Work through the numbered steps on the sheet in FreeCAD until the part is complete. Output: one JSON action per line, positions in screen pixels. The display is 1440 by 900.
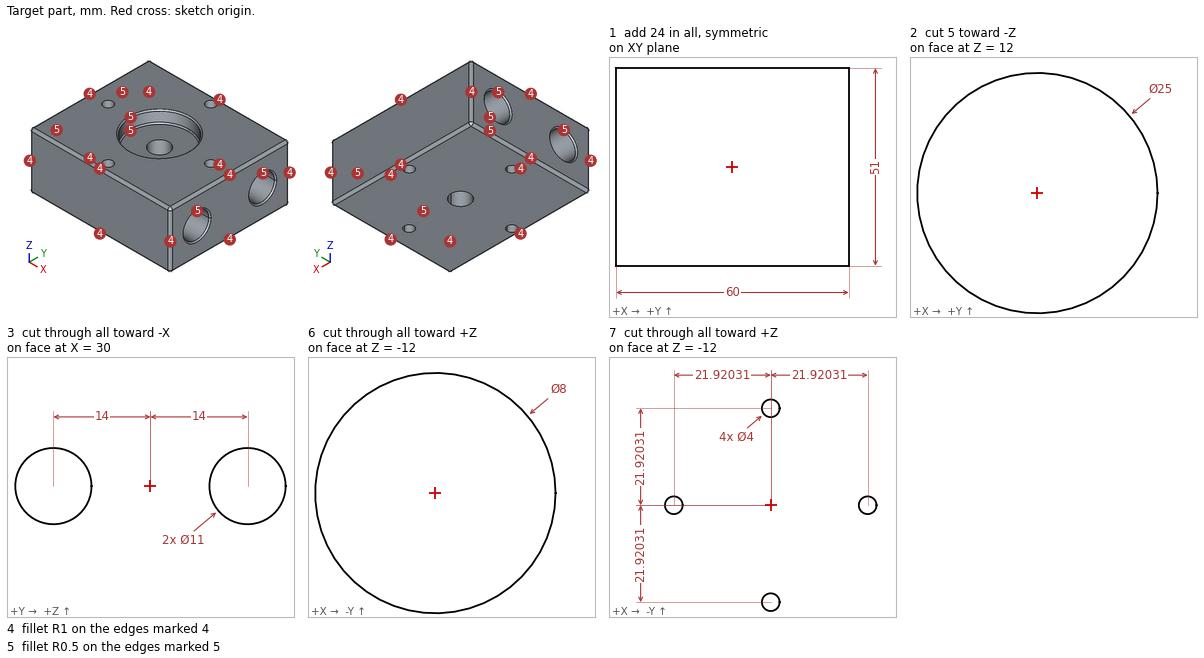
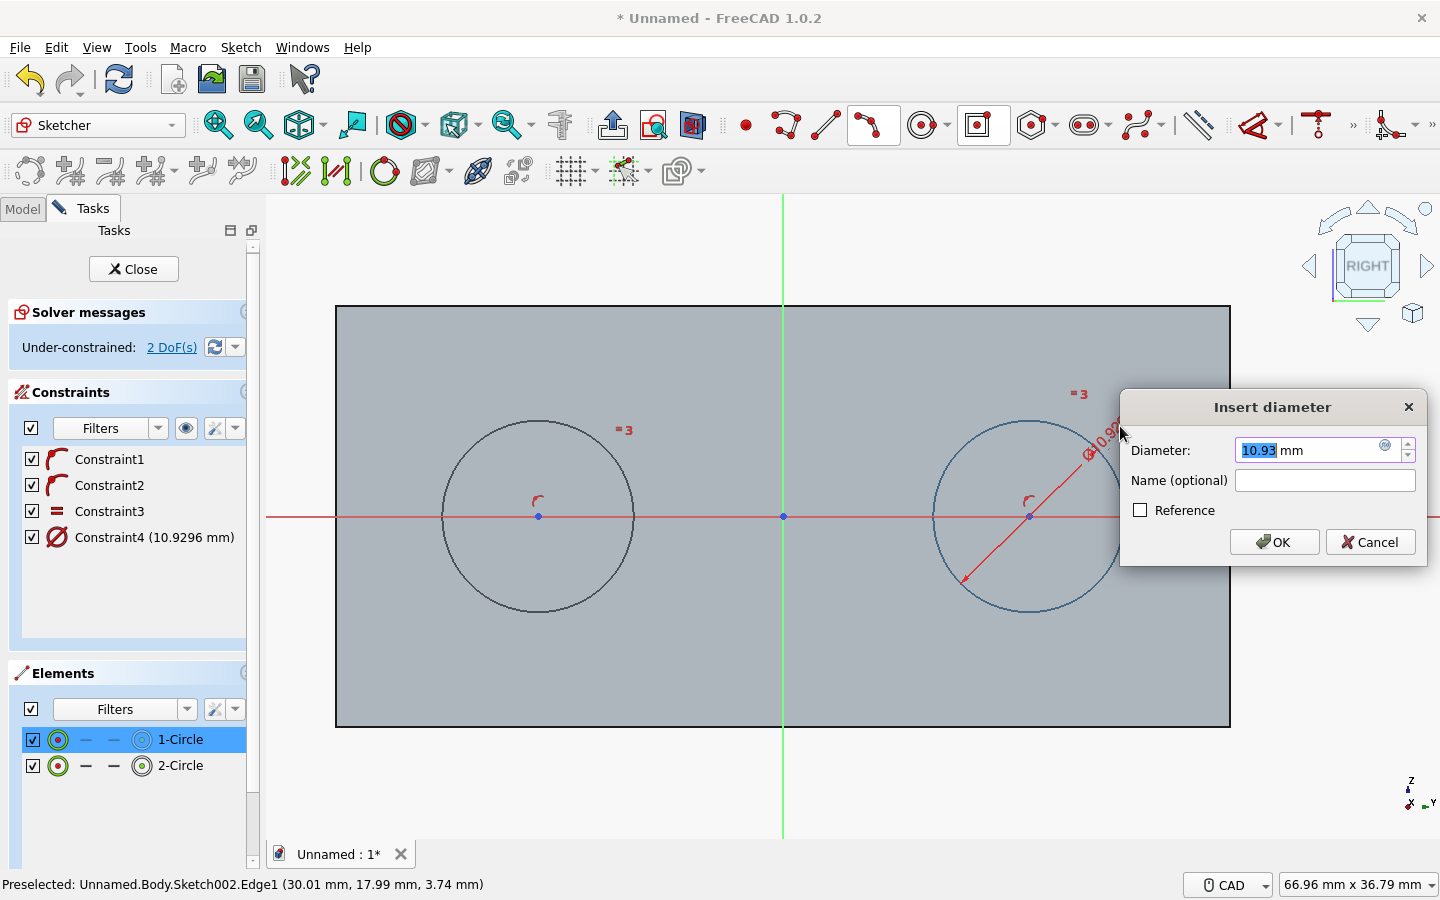
{"action": "type", "text": "11"}
{"action": "key", "text": "Return"}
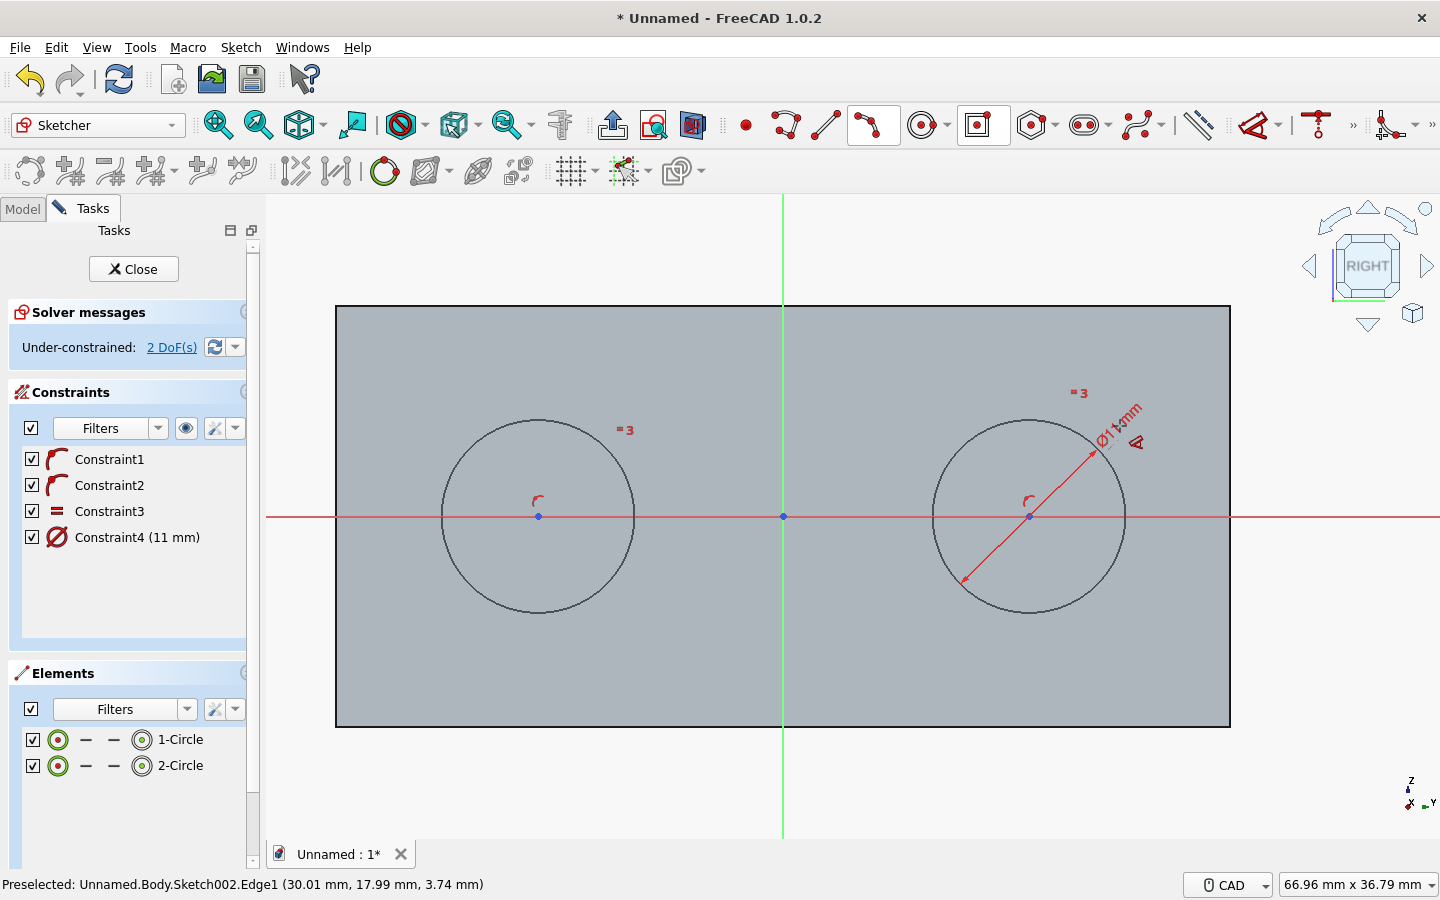
{"action": "left_click", "coordinate": [1029, 516]}
{"action": "left_click", "coordinate": [906, 550]}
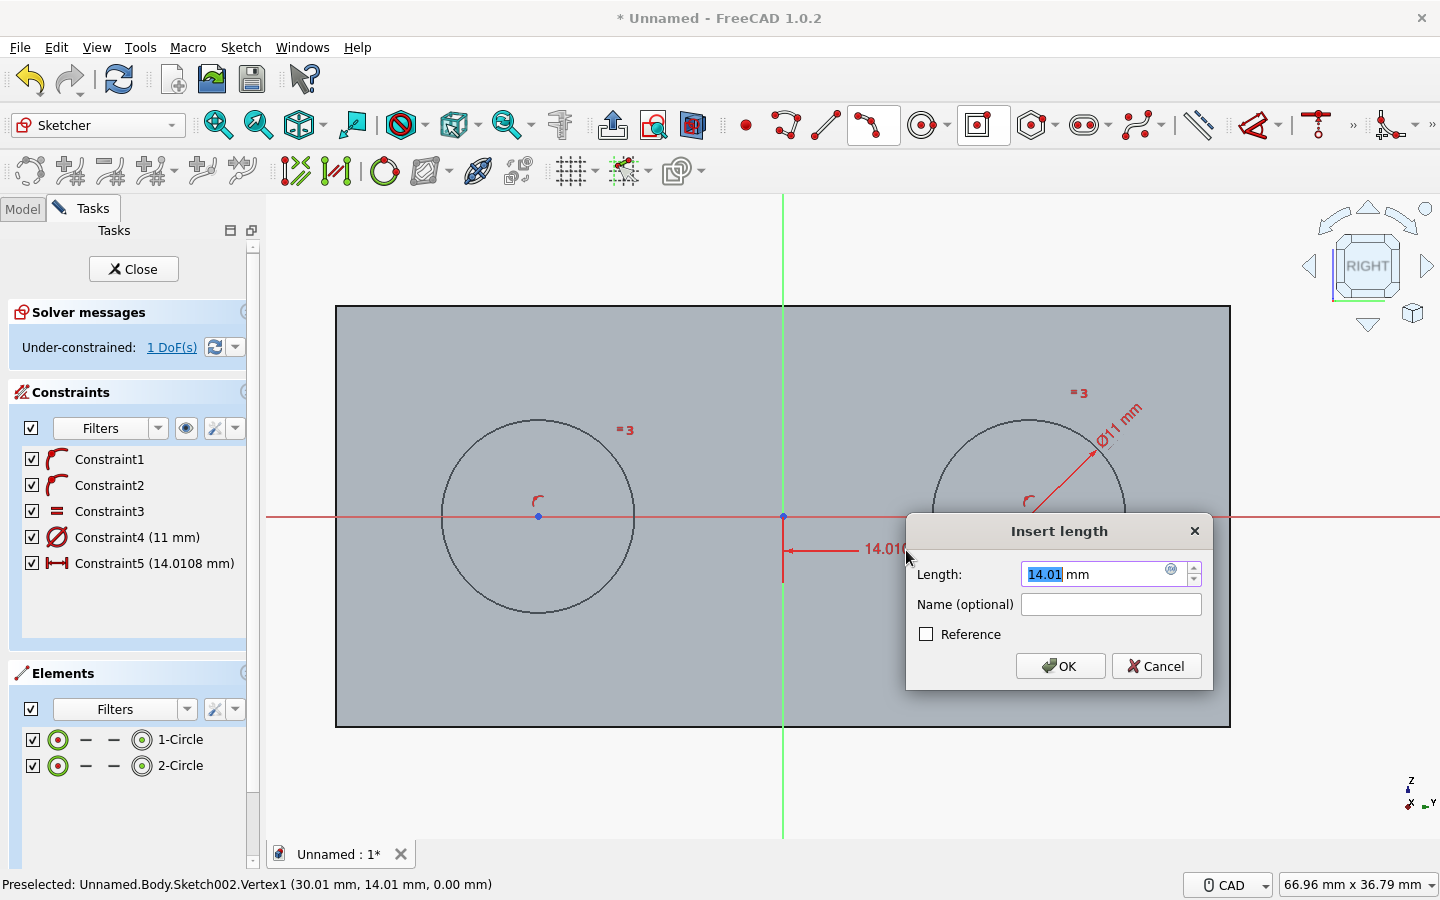
{"action": "type", "text": "14"}
{"action": "key", "text": "Return"}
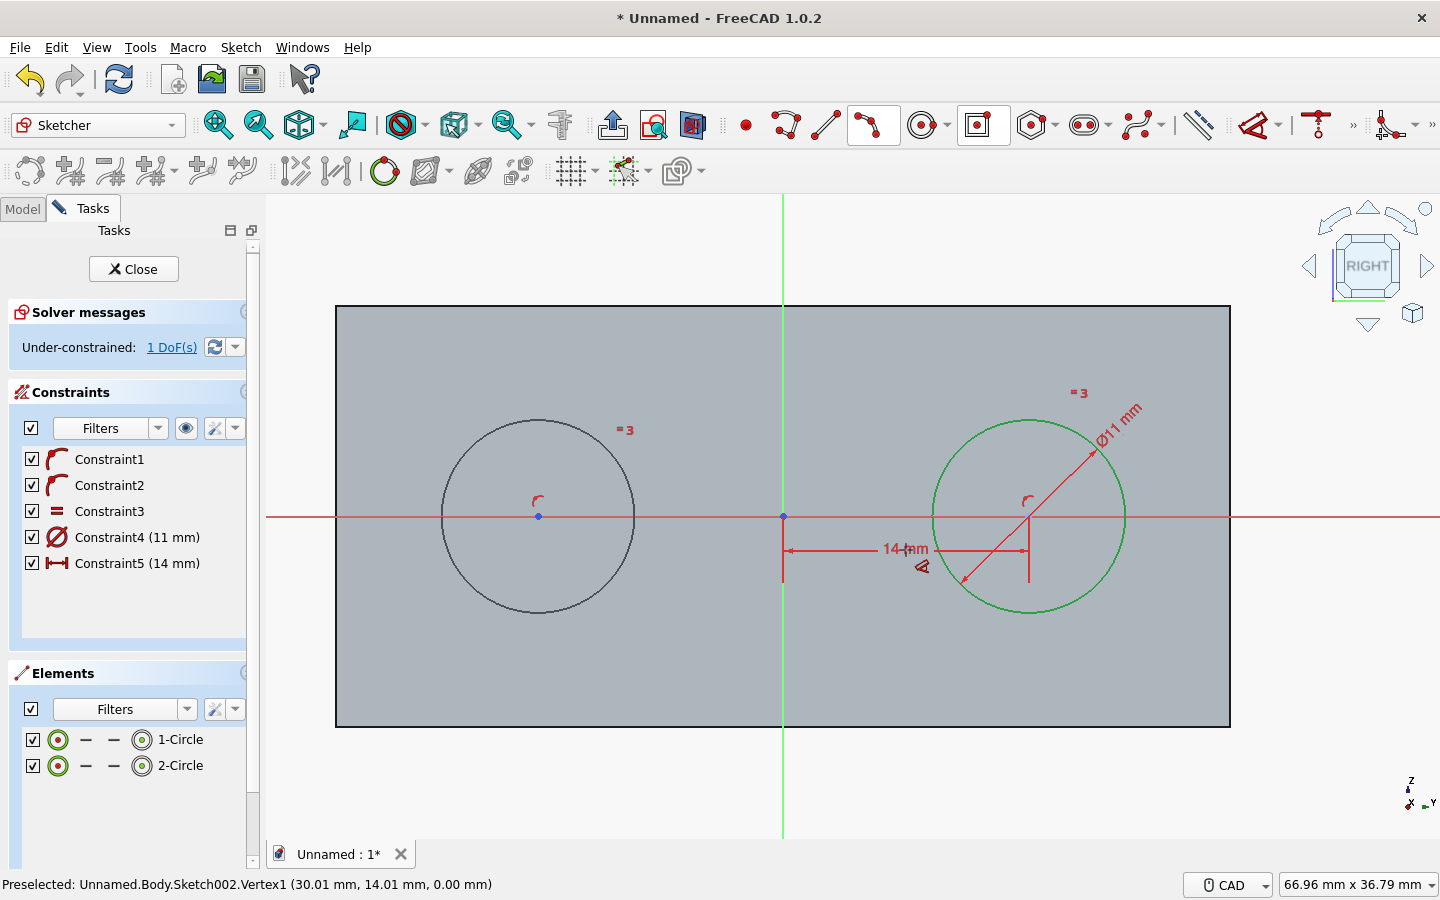
{"action": "left_click", "coordinate": [538, 516]}
{"action": "left_click", "coordinate": [661, 550]}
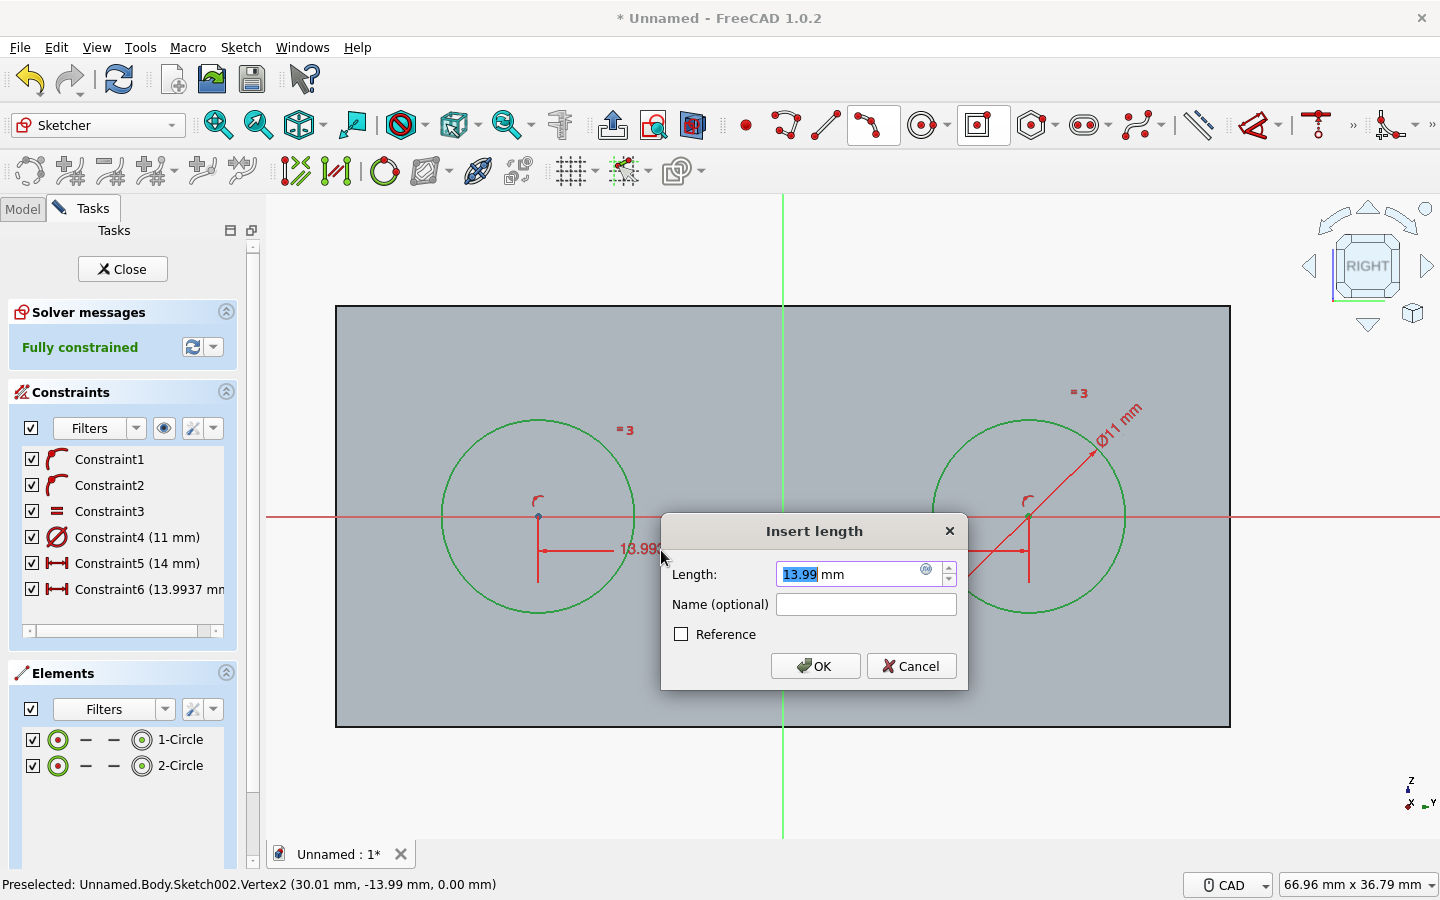
{"action": "type", "text": "14"}
{"action": "key", "text": "Return"}
{"action": "key", "text": "Escape"}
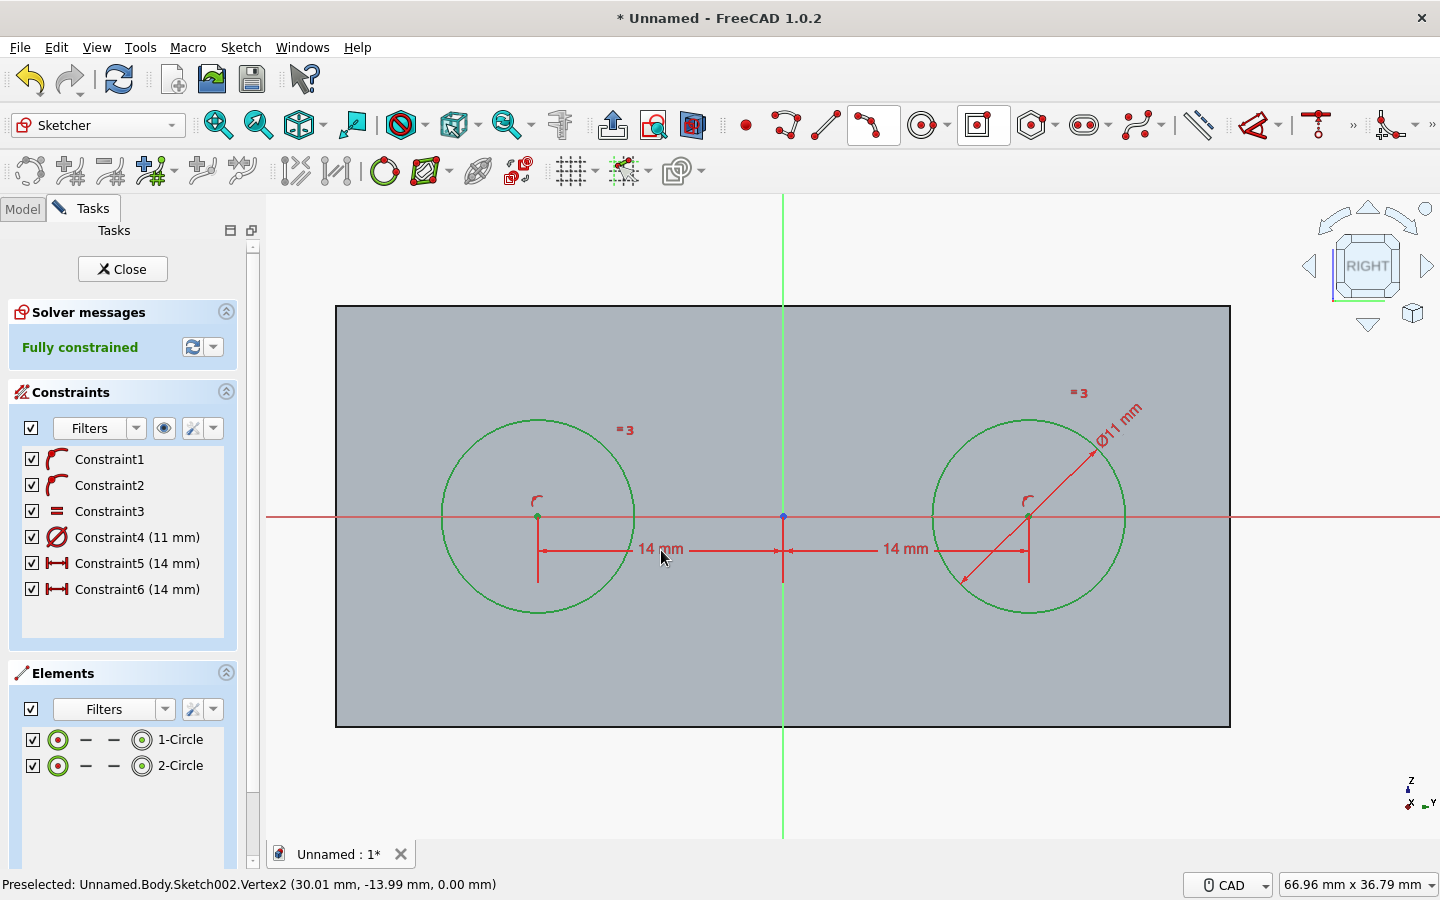
{"action": "left_click", "coordinate": [123, 269]}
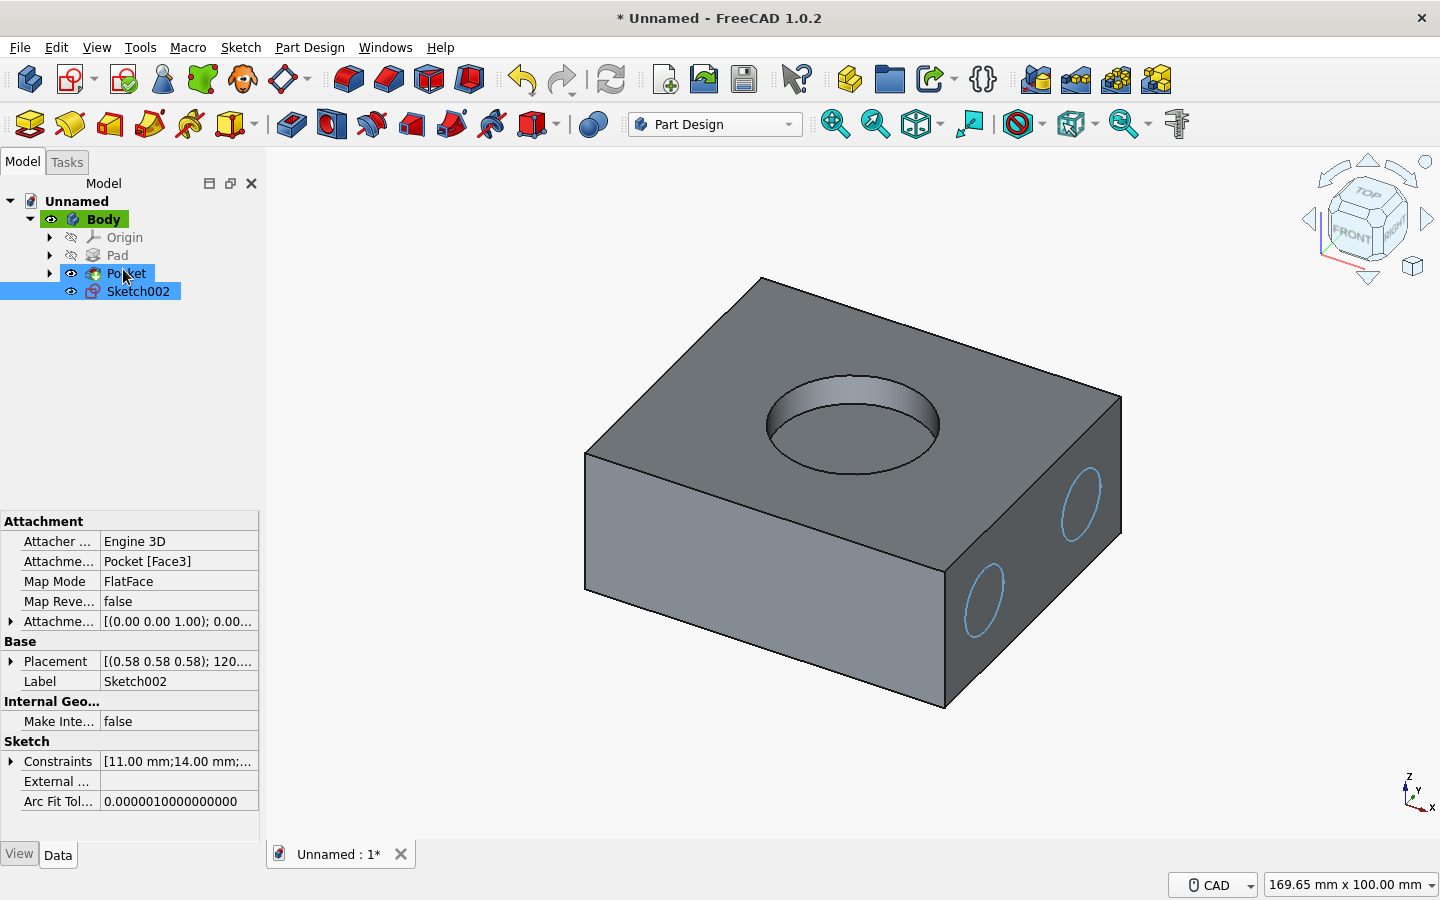
{"action": "left_click", "coordinate": [292, 124]}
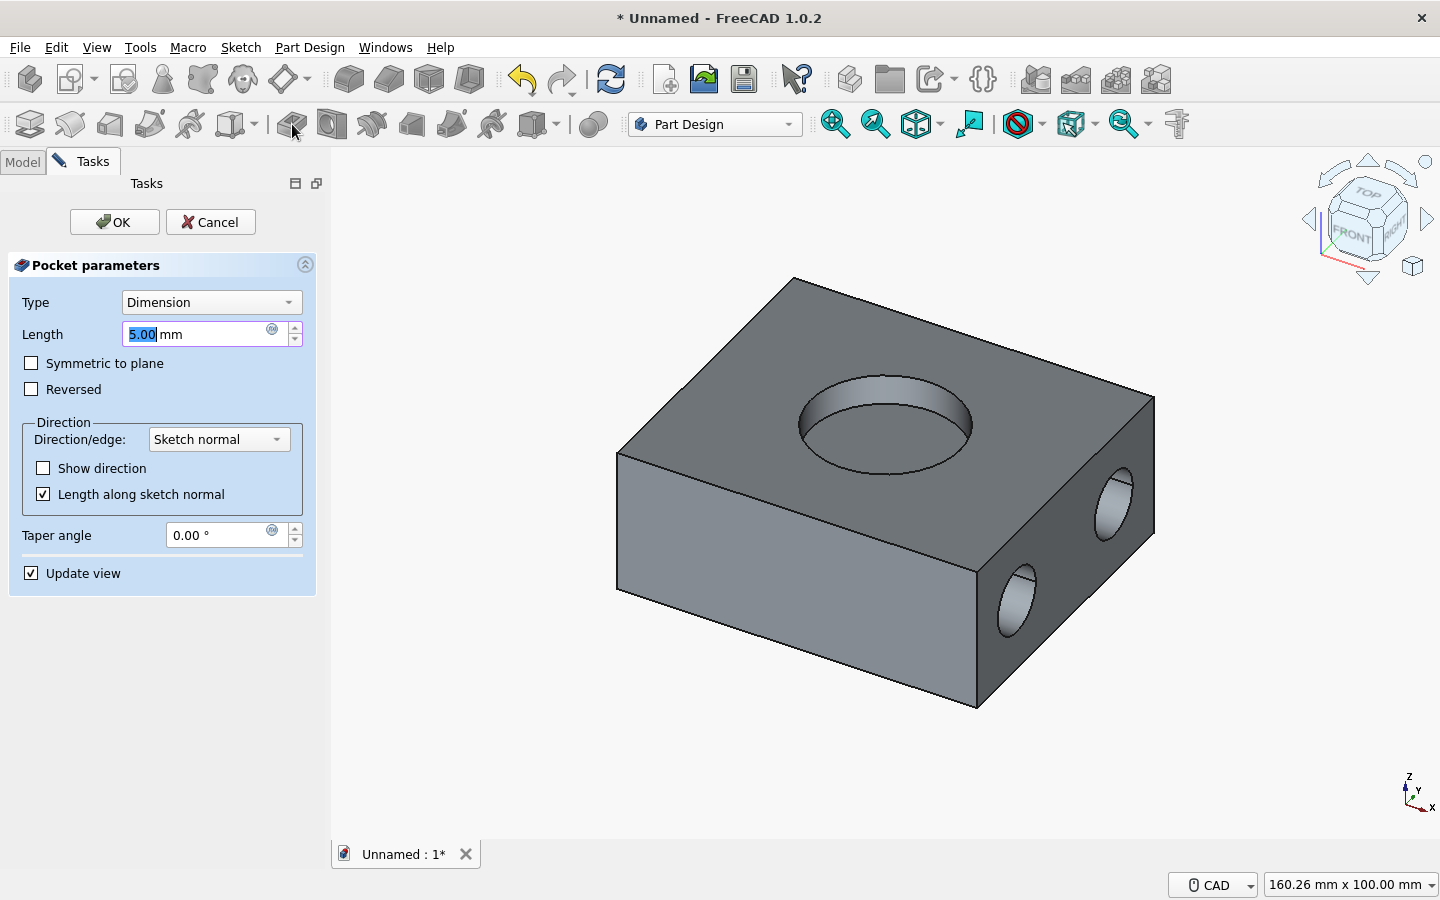
{"action": "left_click", "coordinate": [212, 302]}